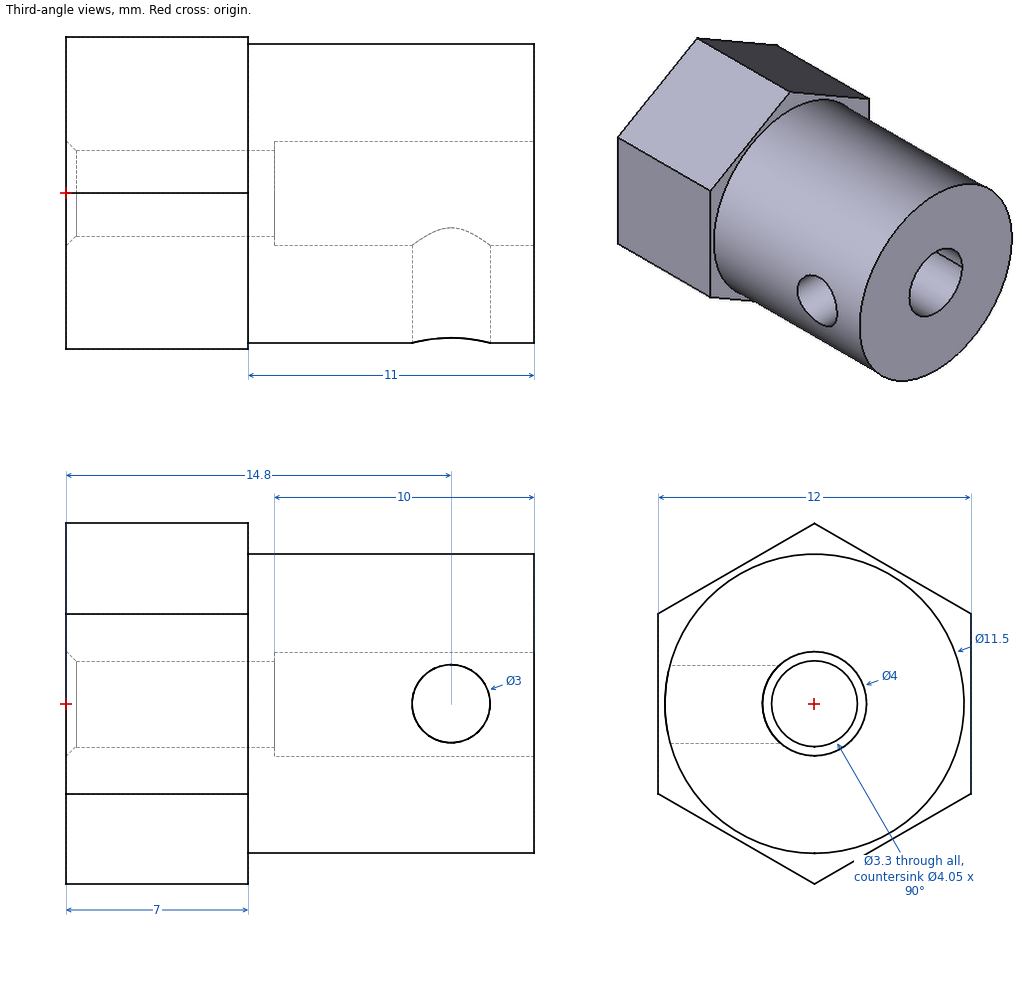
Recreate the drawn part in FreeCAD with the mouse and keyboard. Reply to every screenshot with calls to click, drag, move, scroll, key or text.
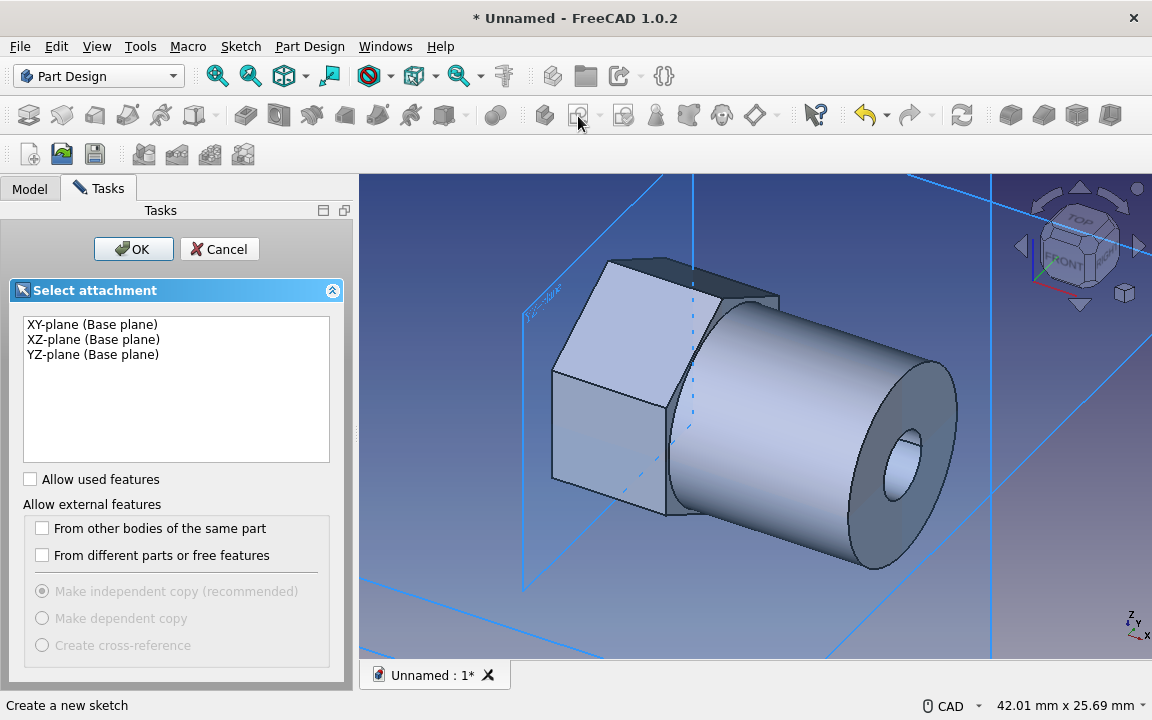
click(84, 340)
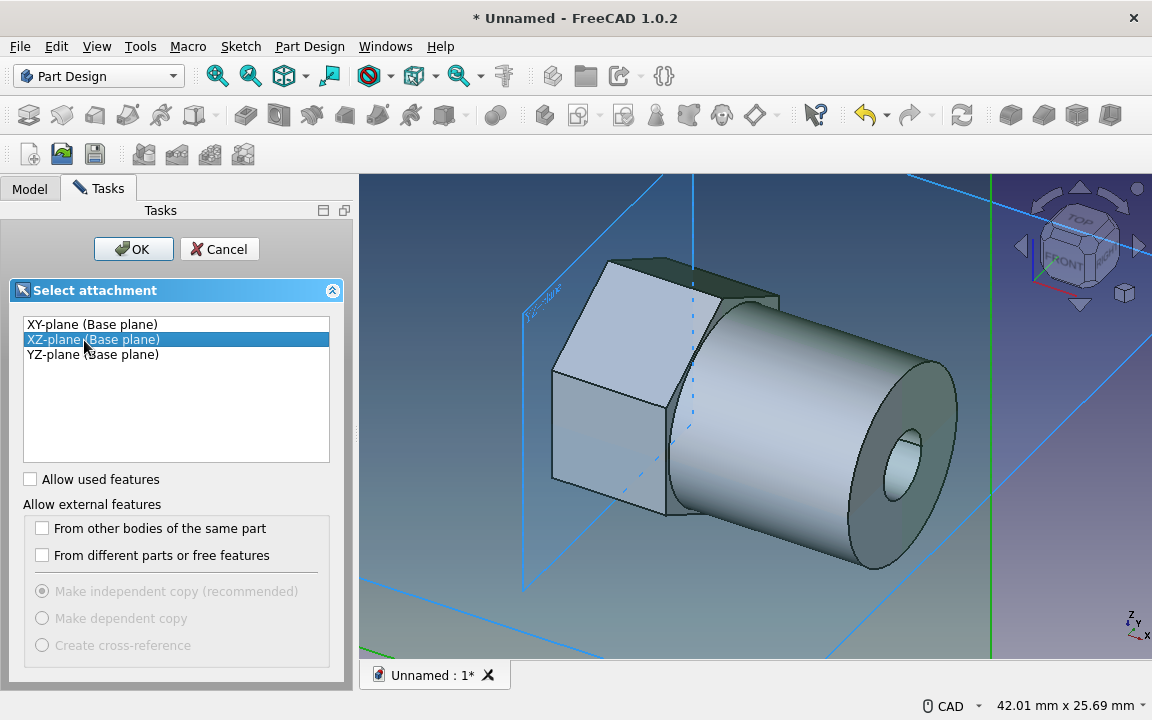
click(134, 249)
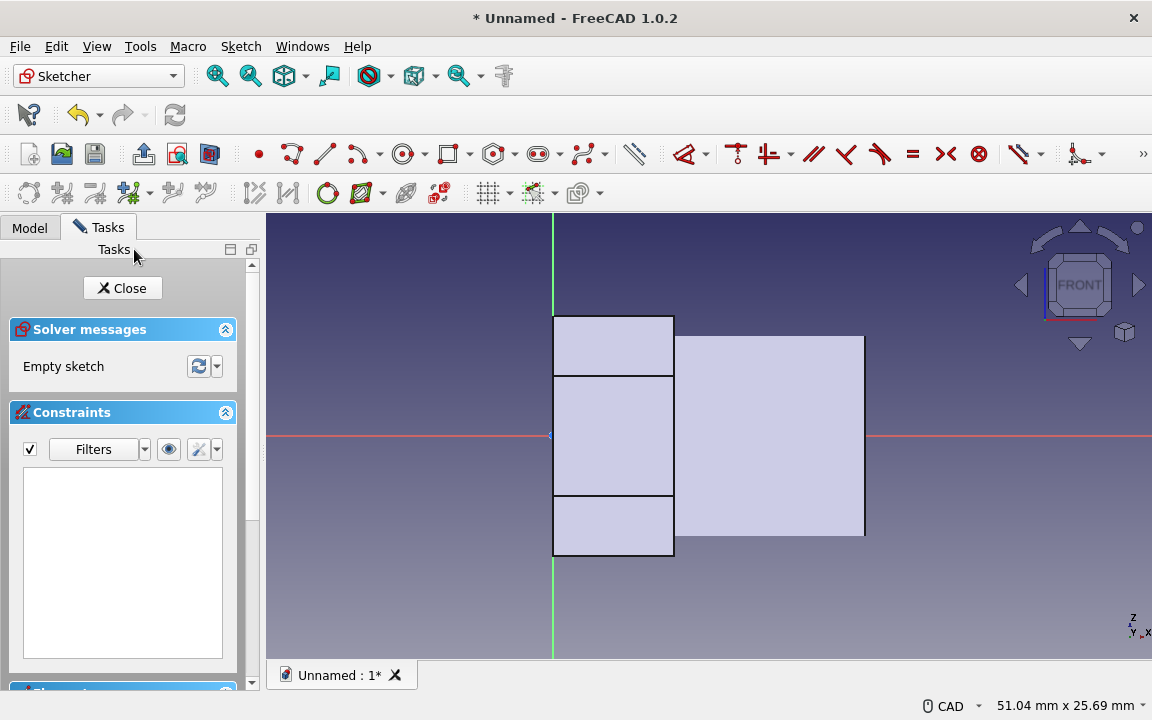
key(q)
key(s)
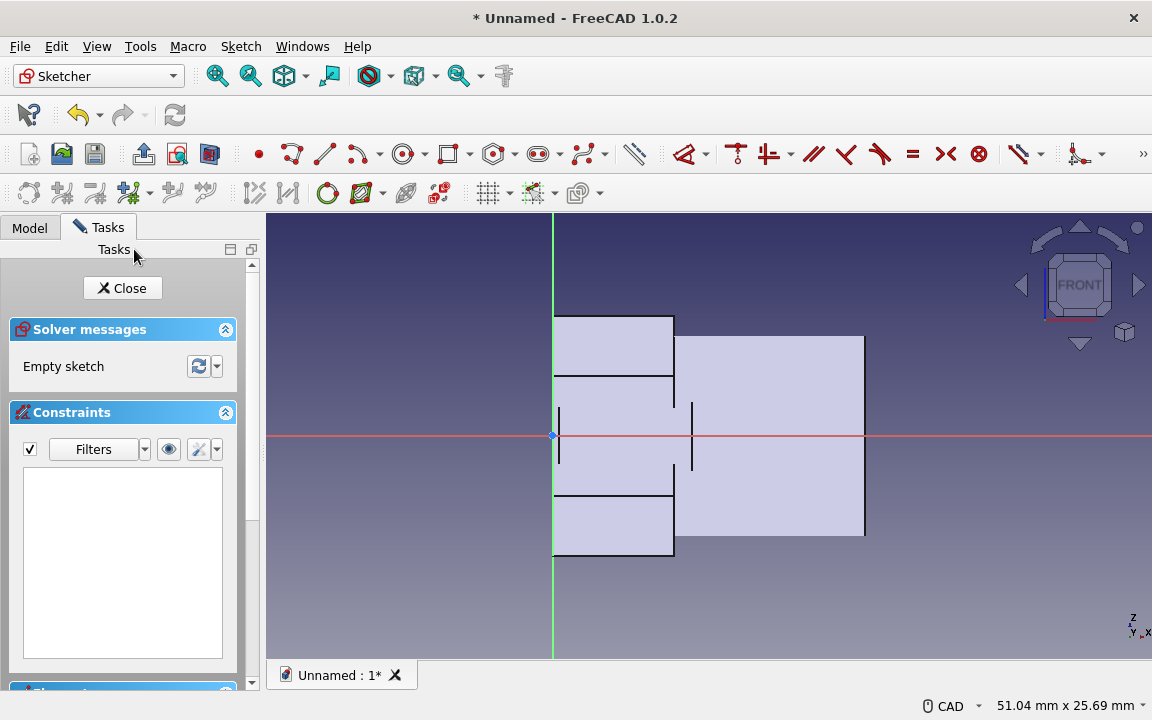
scroll(852, 436, up, 8)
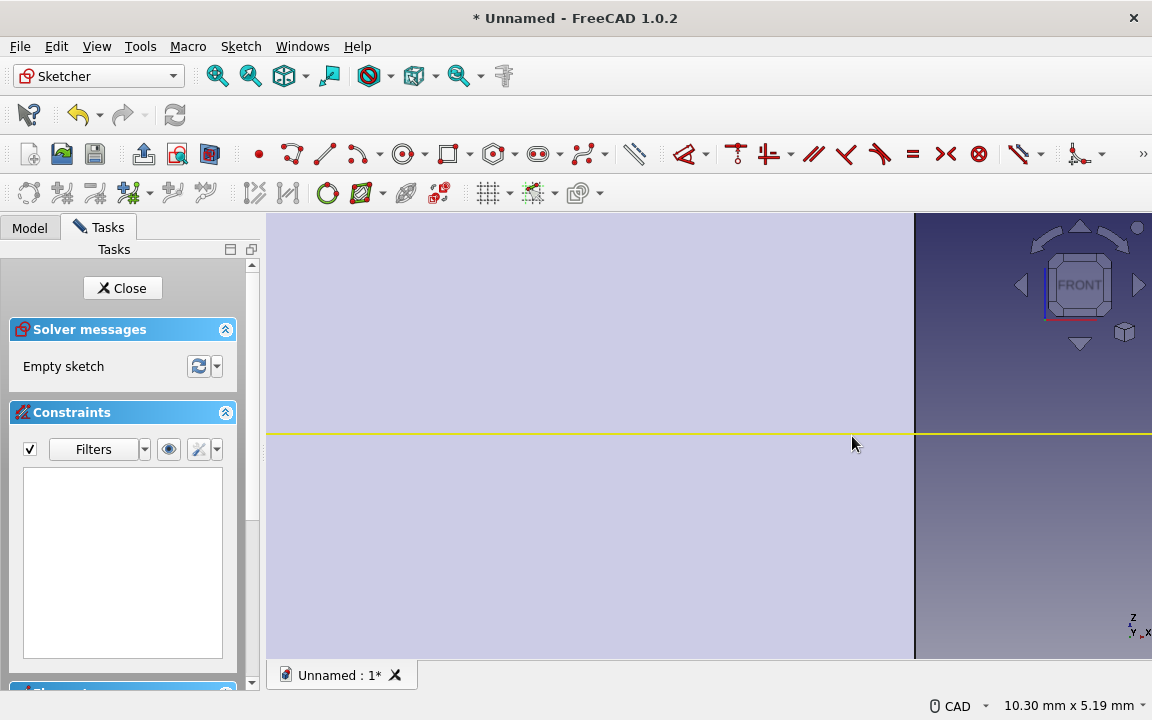
key(g)
key(c)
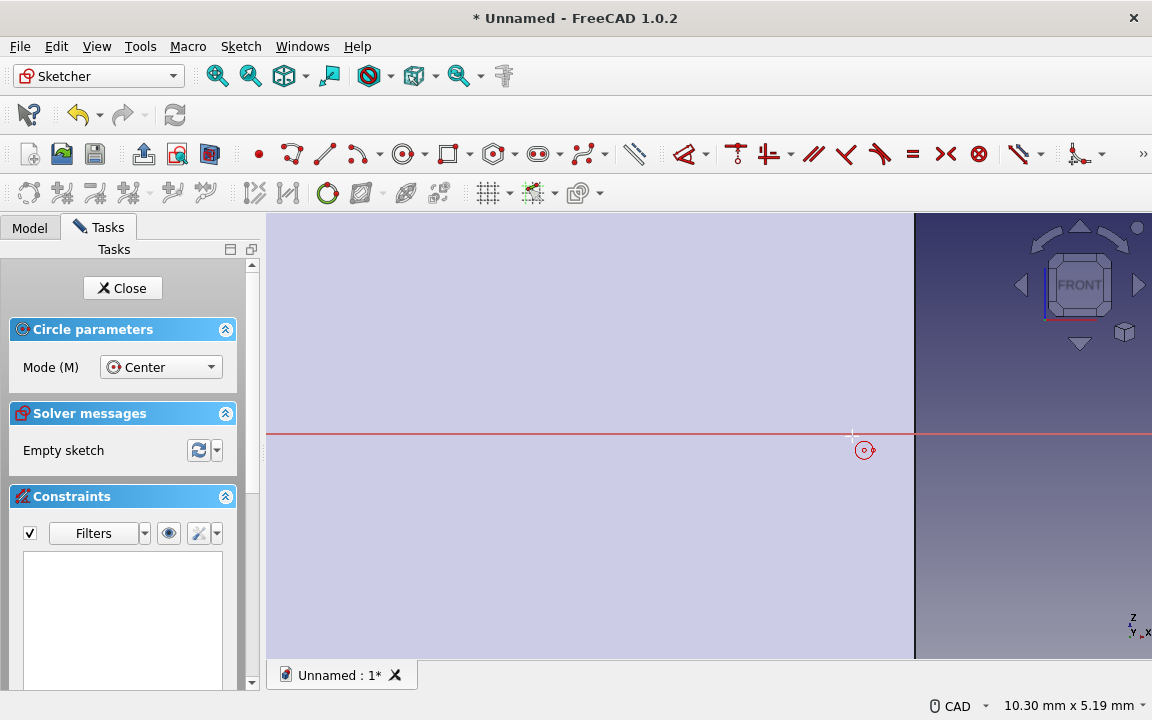
click(640, 434)
move(731, 343)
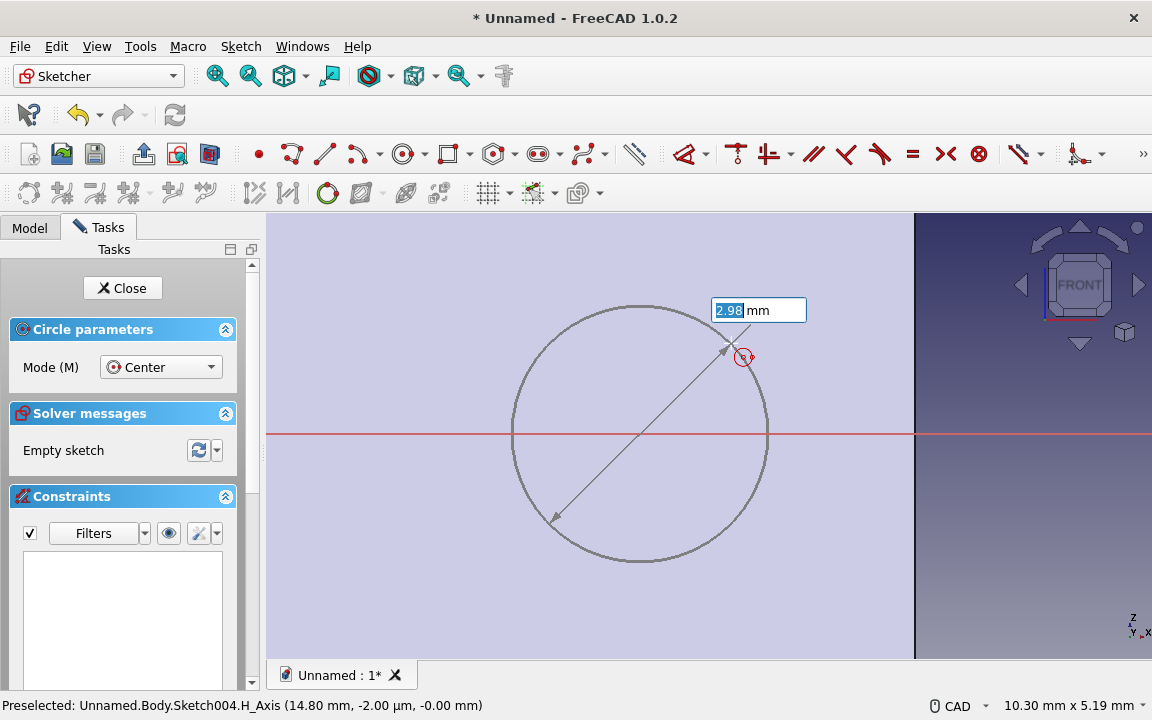
text(3)
key(Return)
key(Escape)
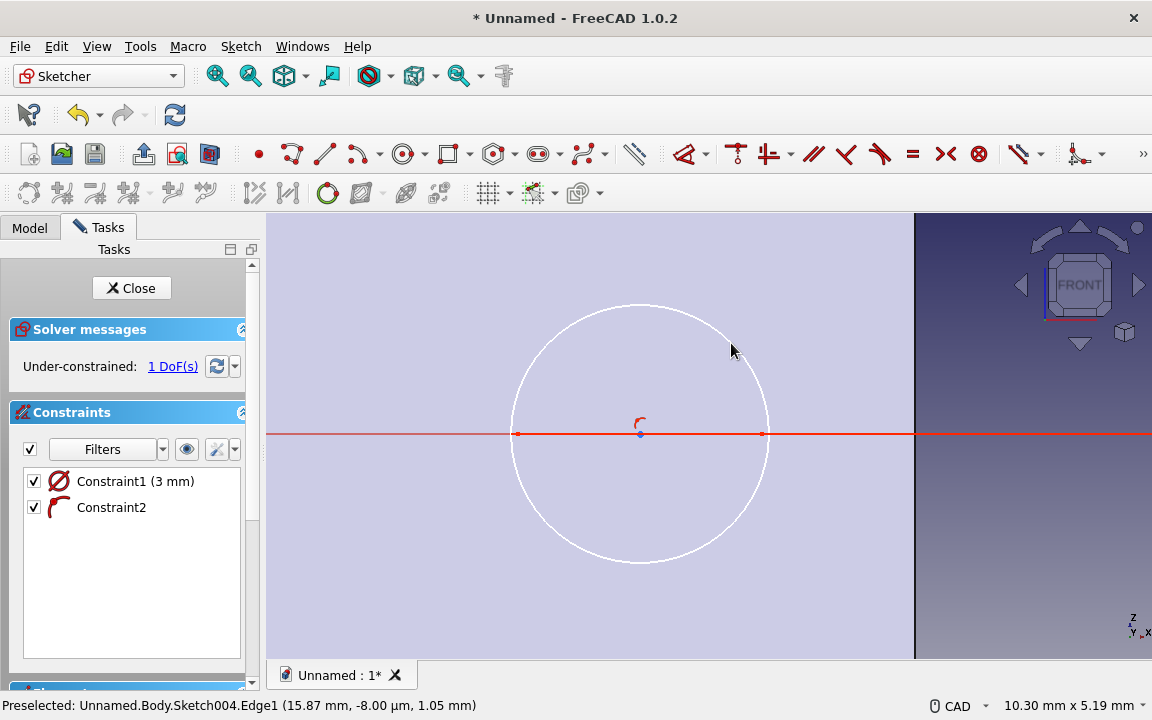
key(d)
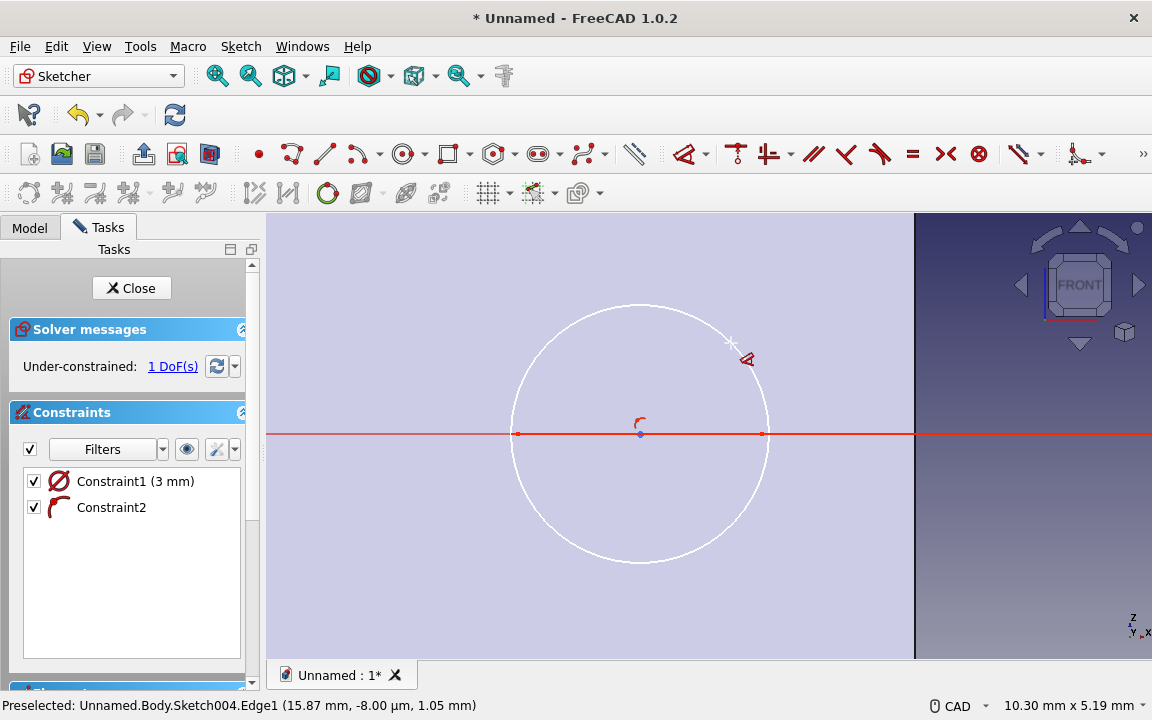
click(640, 434)
click(467, 468)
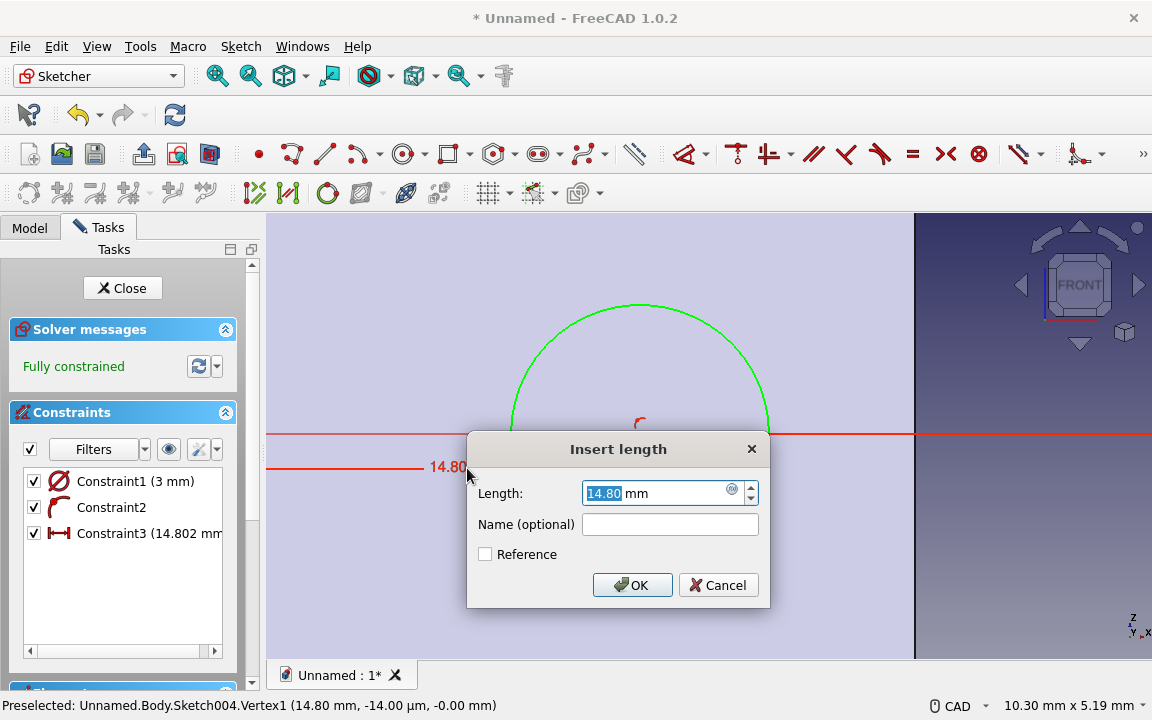
text(14.8)
key(Return)
key(Escape)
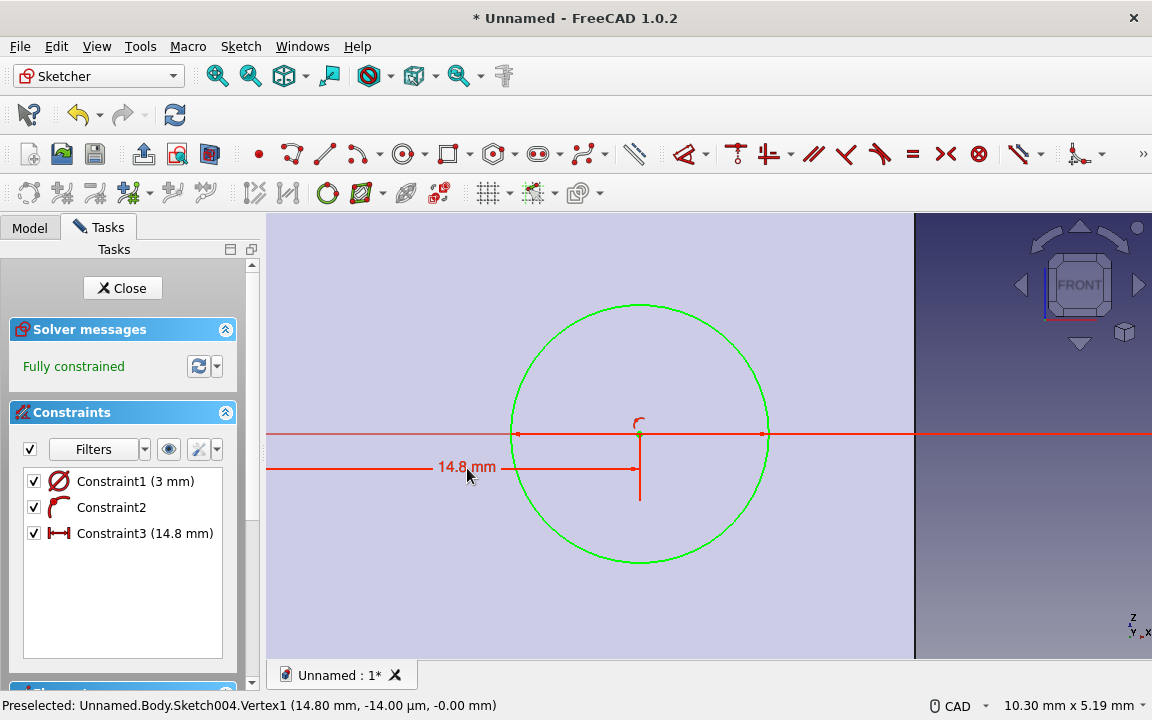
click(123, 288)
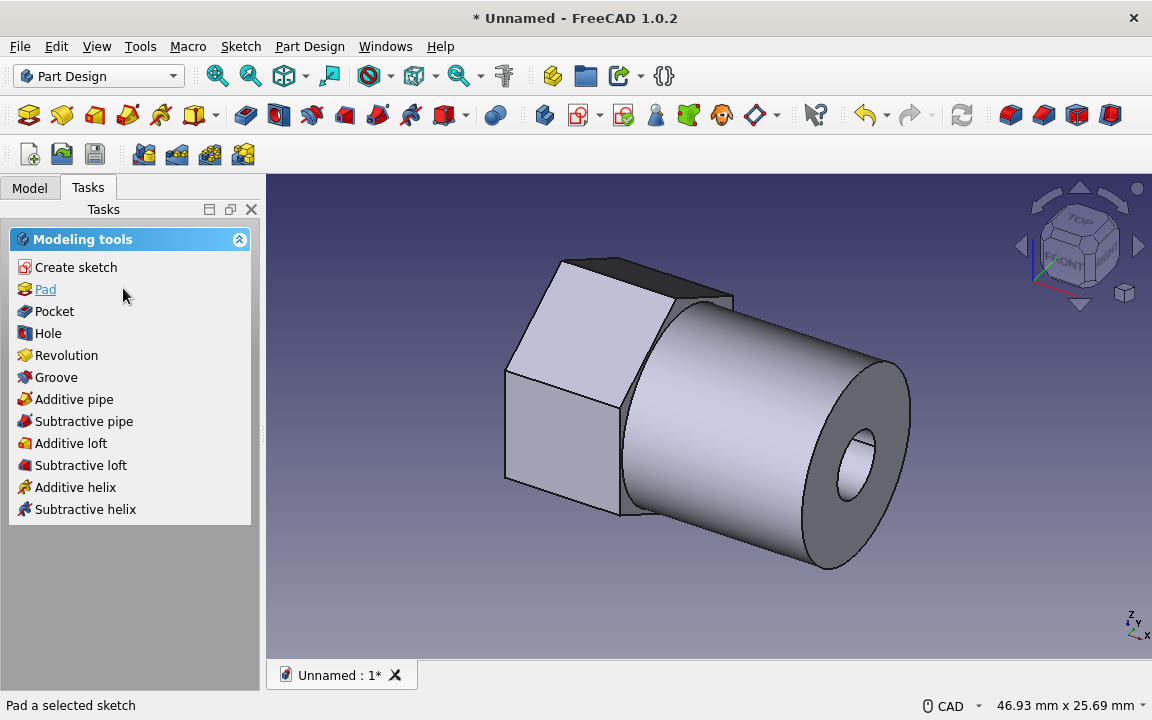
click(246, 116)